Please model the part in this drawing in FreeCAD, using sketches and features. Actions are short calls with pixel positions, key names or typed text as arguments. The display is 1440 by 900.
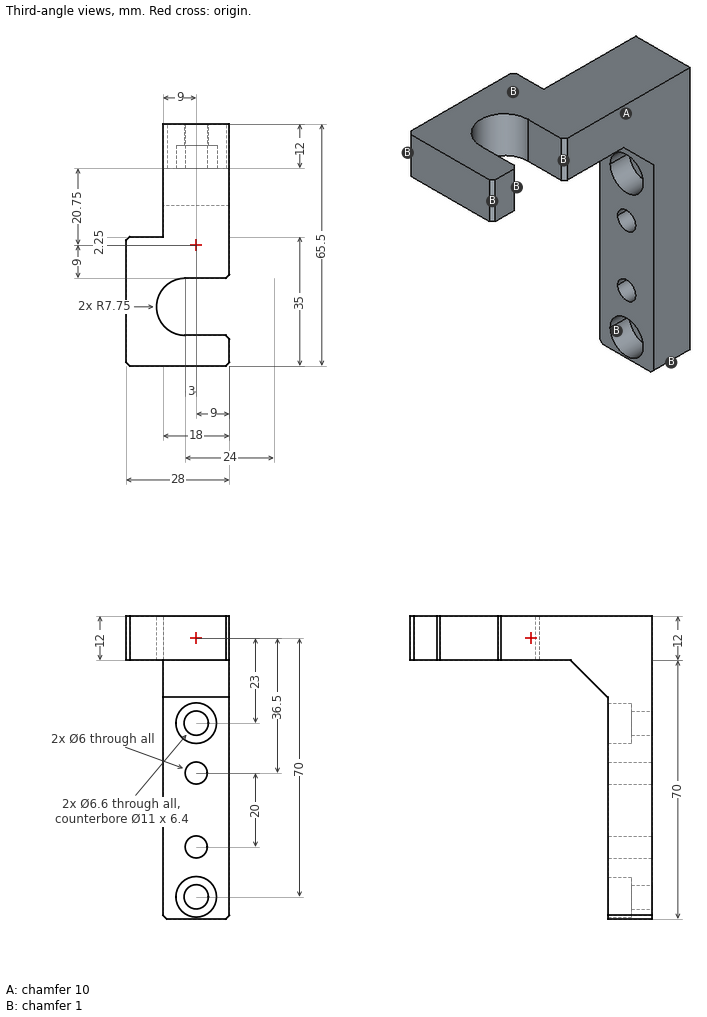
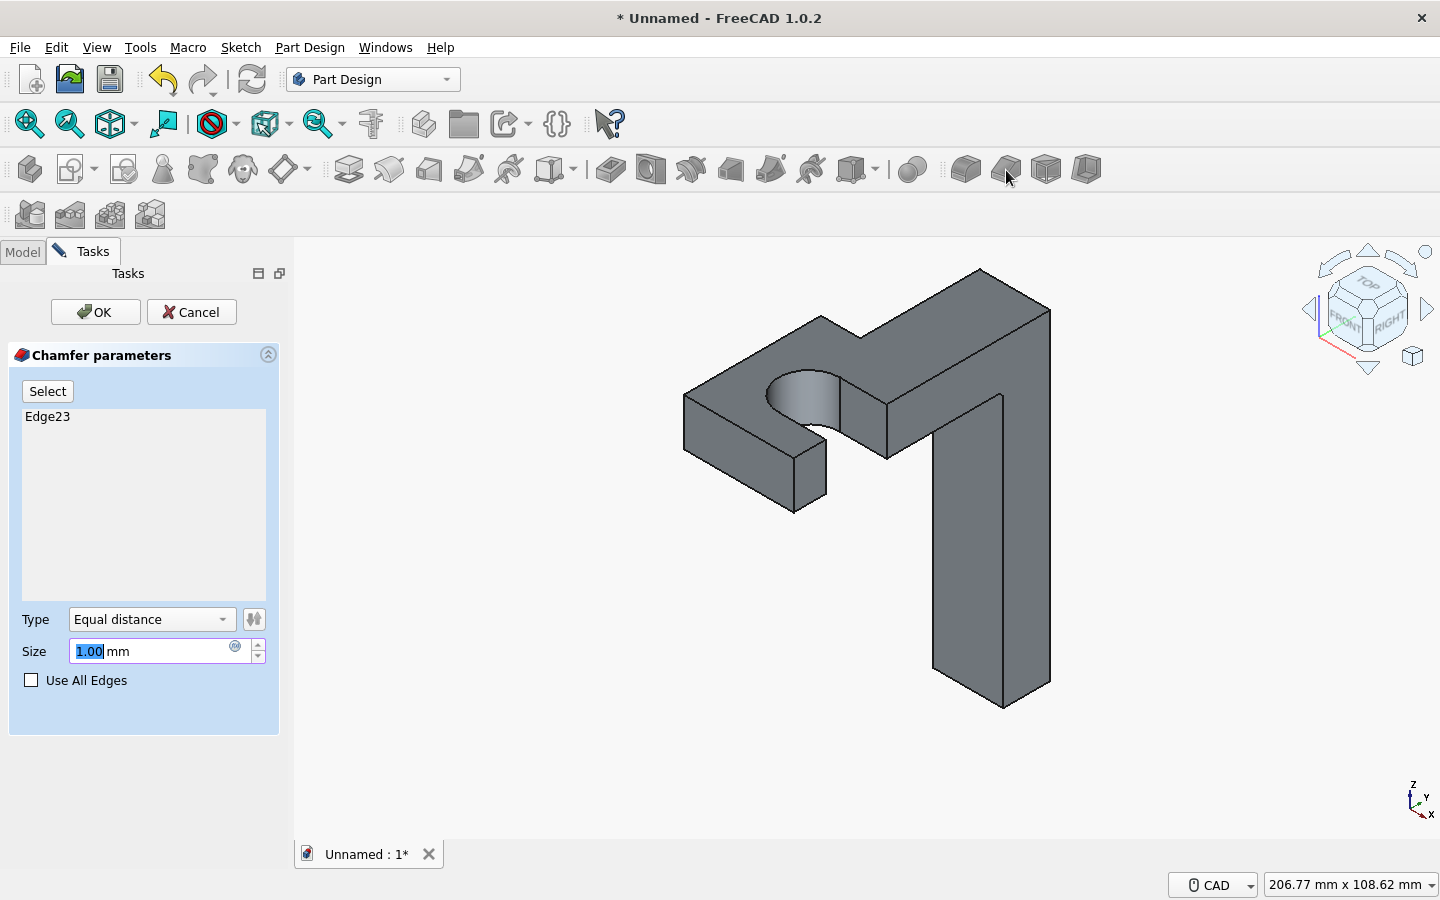
text(10)
key(Tab)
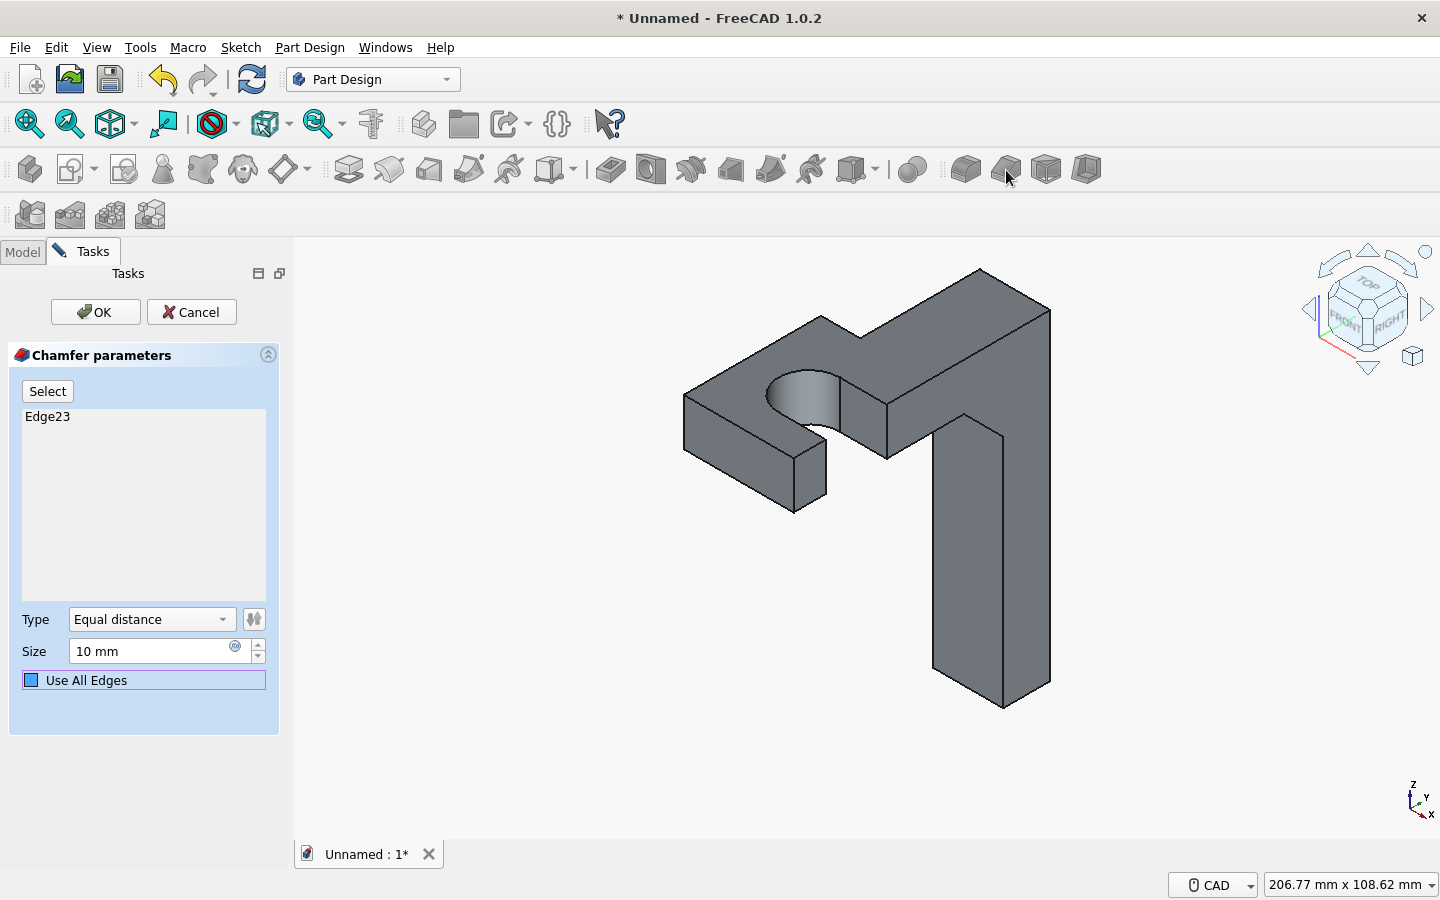
click(96, 312)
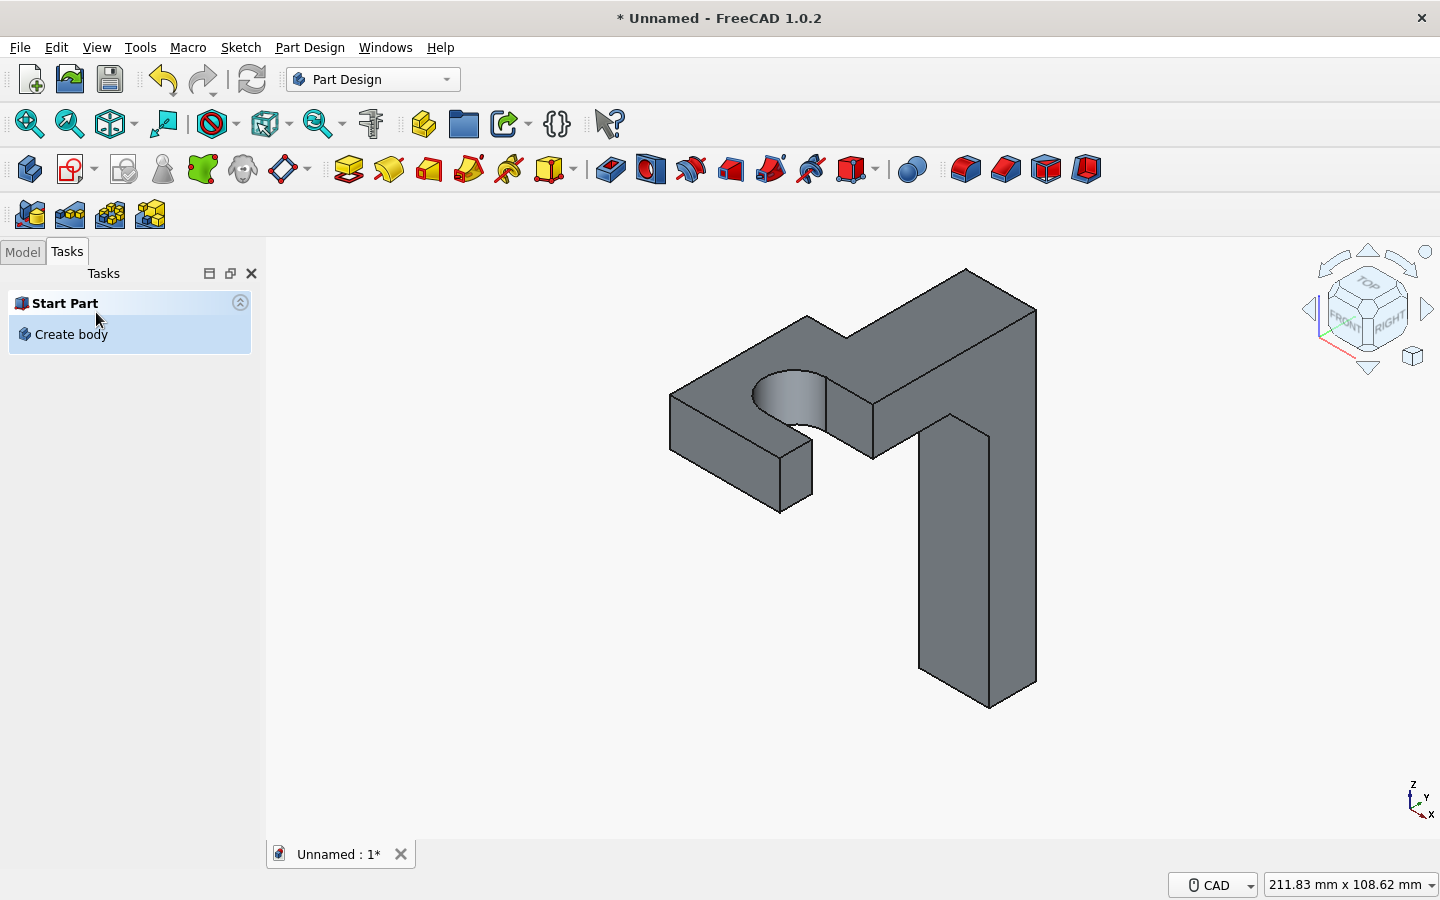
click(954, 474)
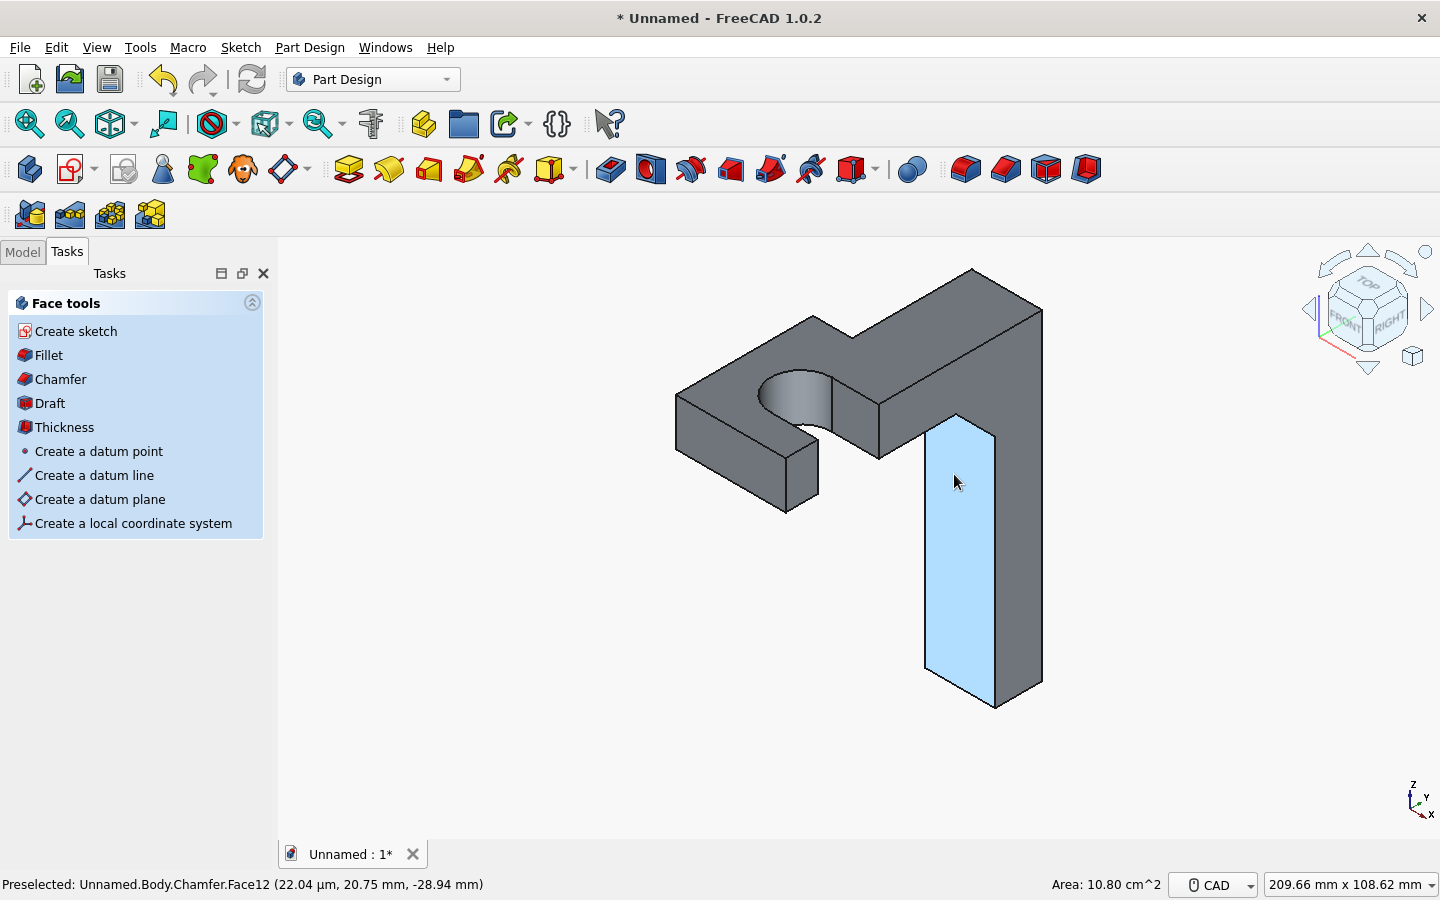
click(70, 170)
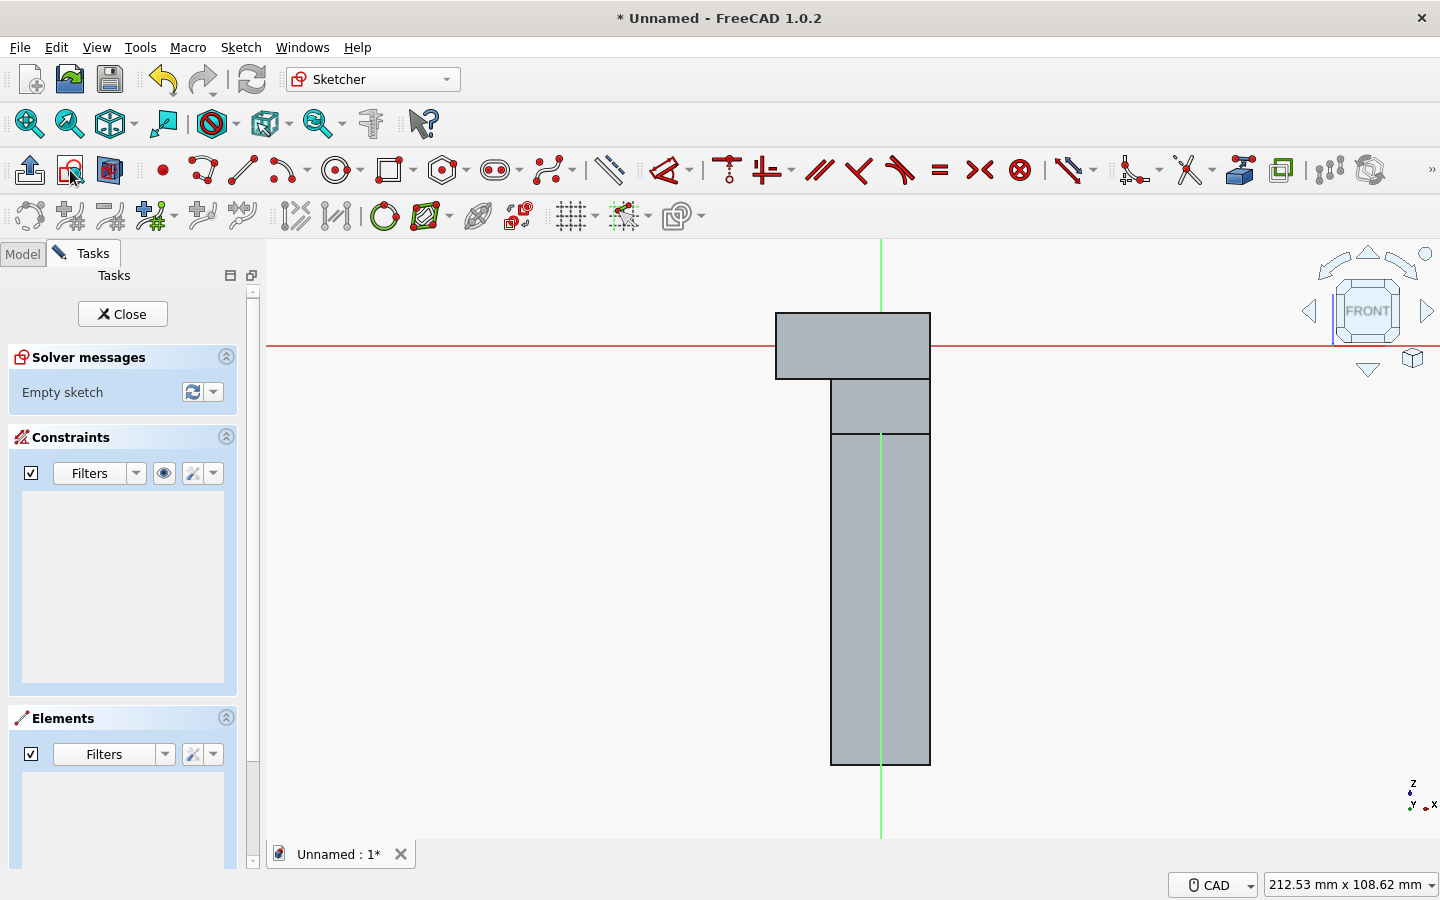
click(336, 170)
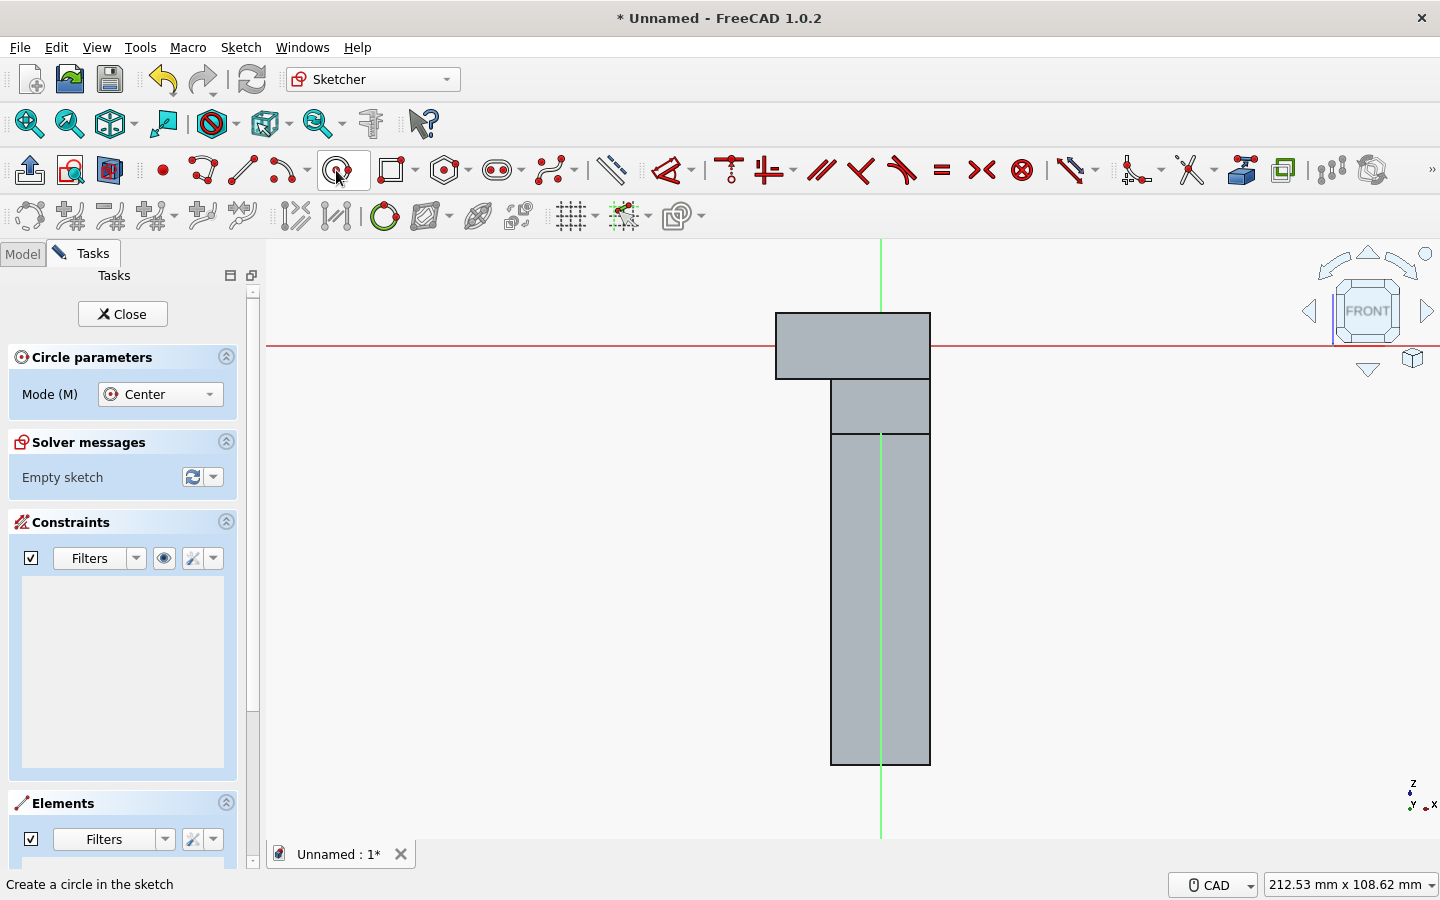
scroll(881, 473, up, 2)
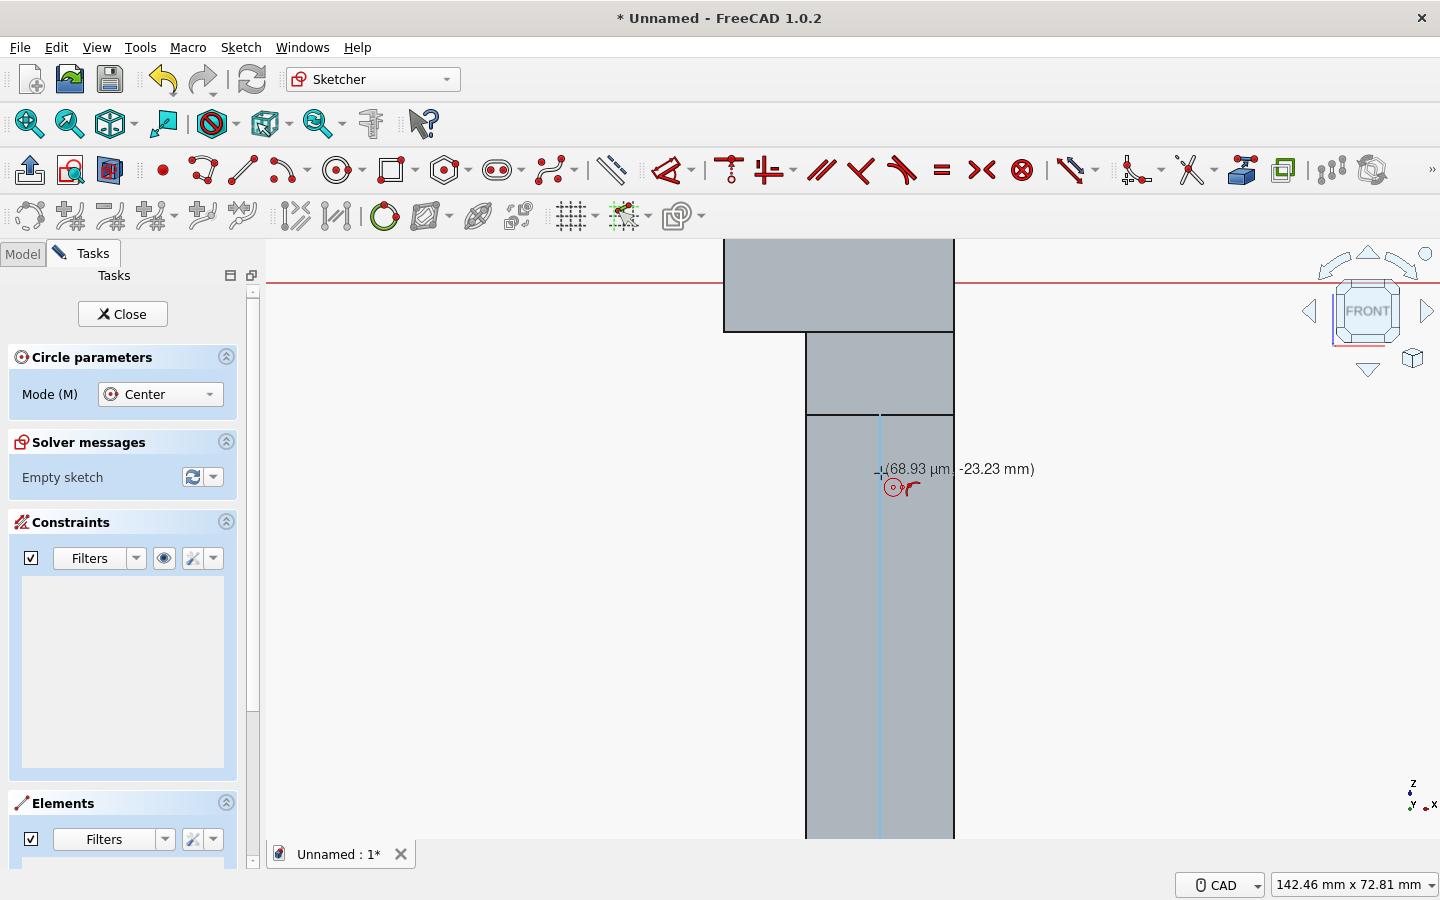
click(880, 472)
move(899, 453)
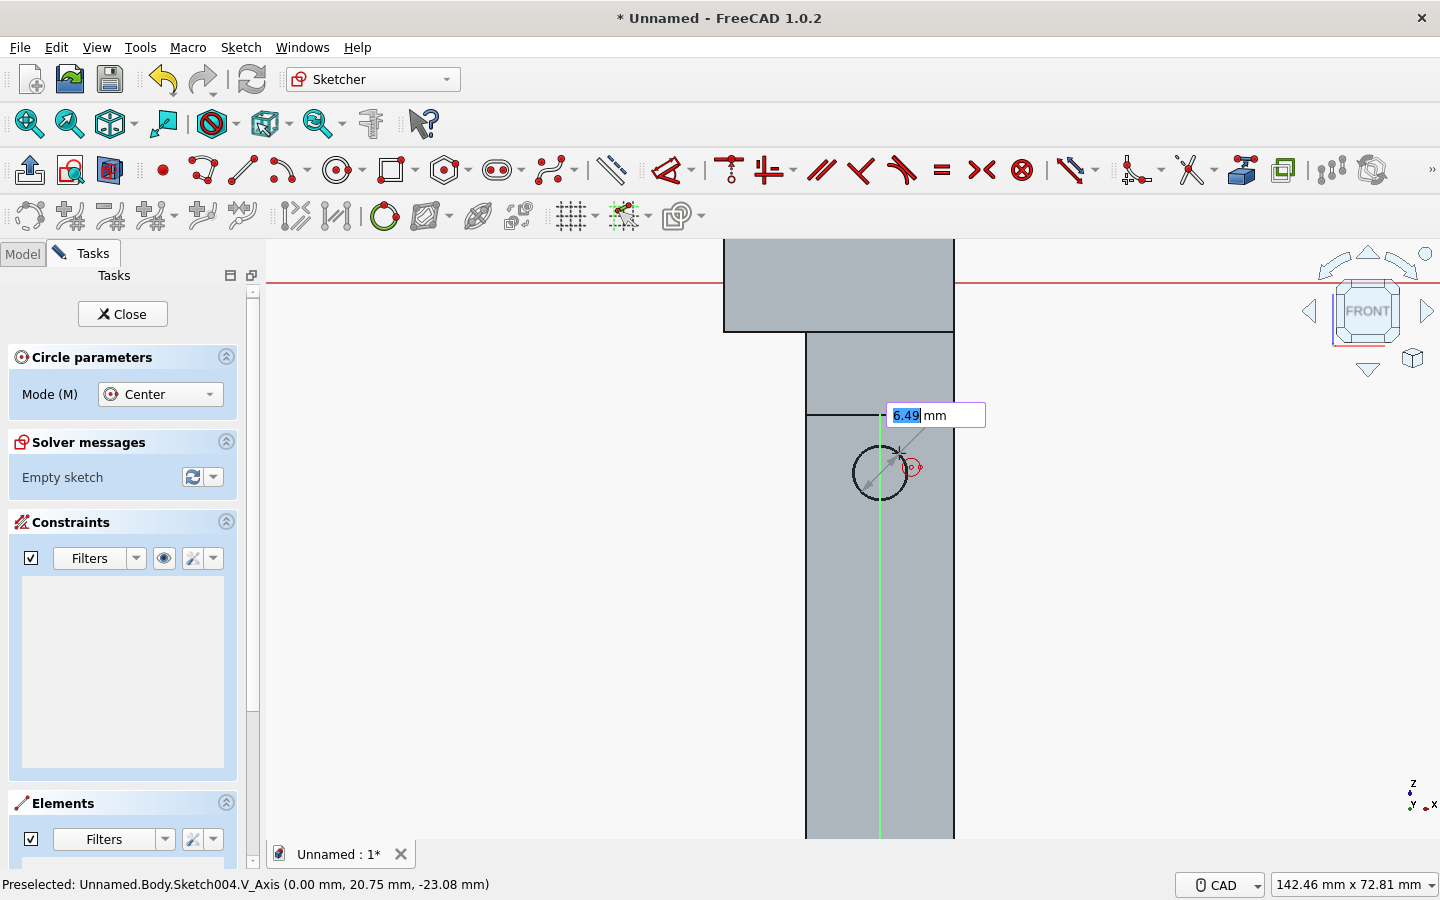
text(6.6)
key(Return)